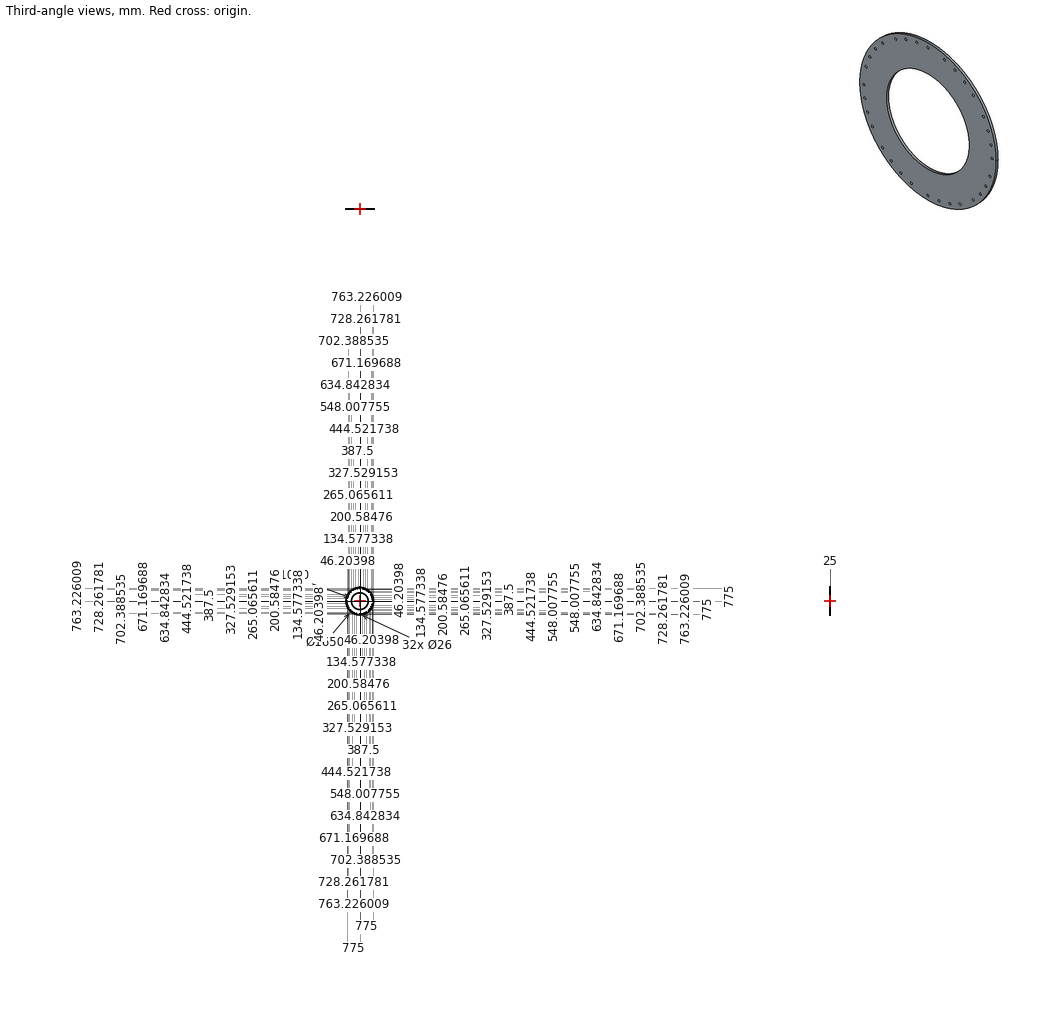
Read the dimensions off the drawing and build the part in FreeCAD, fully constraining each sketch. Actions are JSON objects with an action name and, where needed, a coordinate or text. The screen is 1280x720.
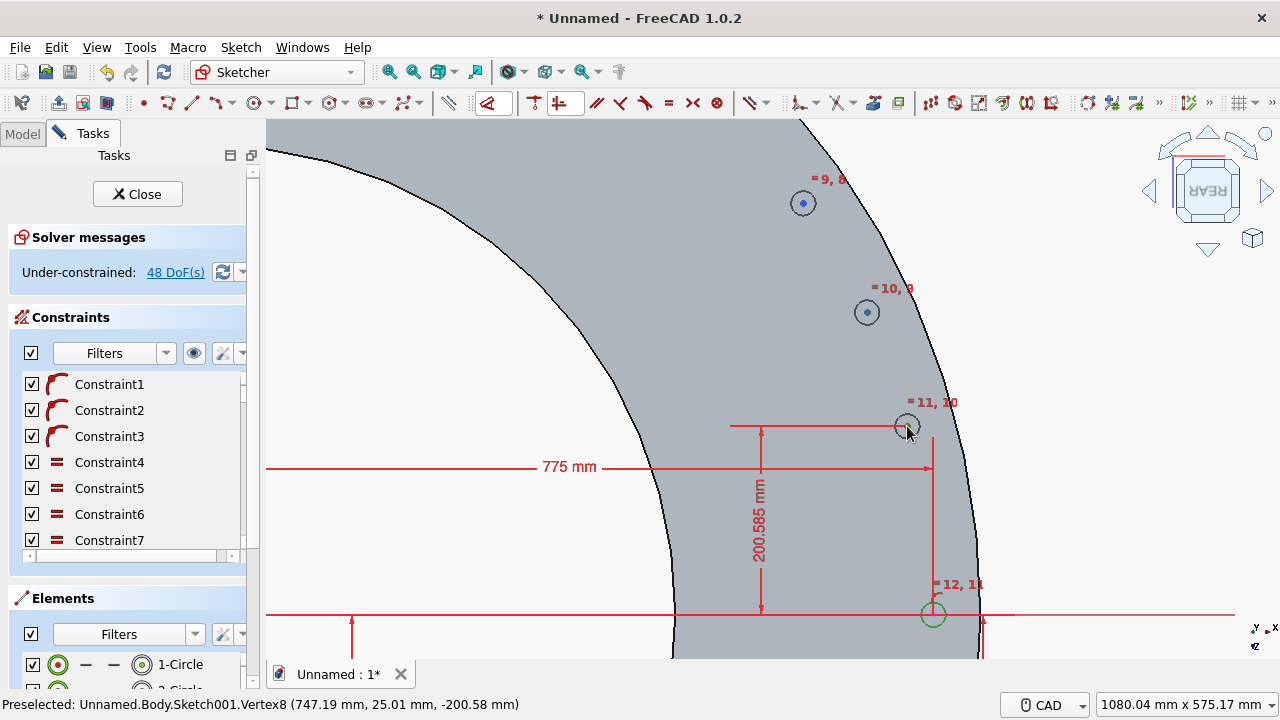
{"action": "key", "text": "l"}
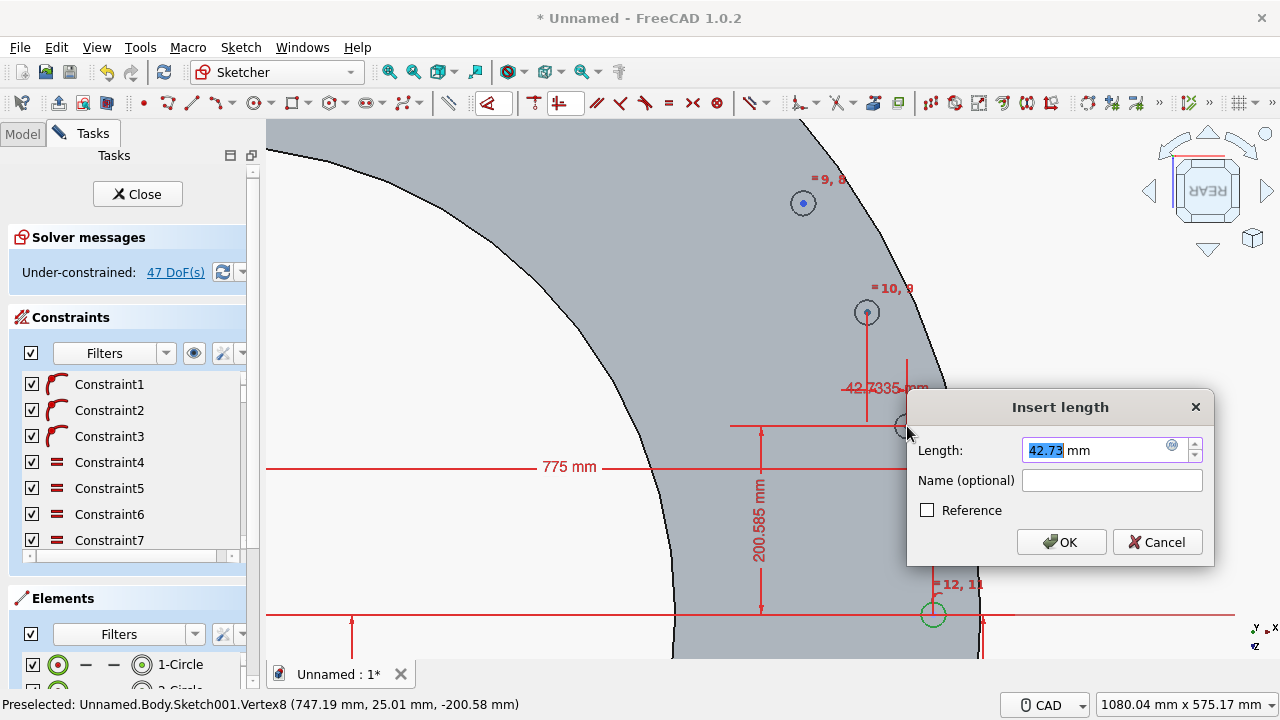
{"action": "type", "text": "46.20398"}
{"action": "key", "text": "Return"}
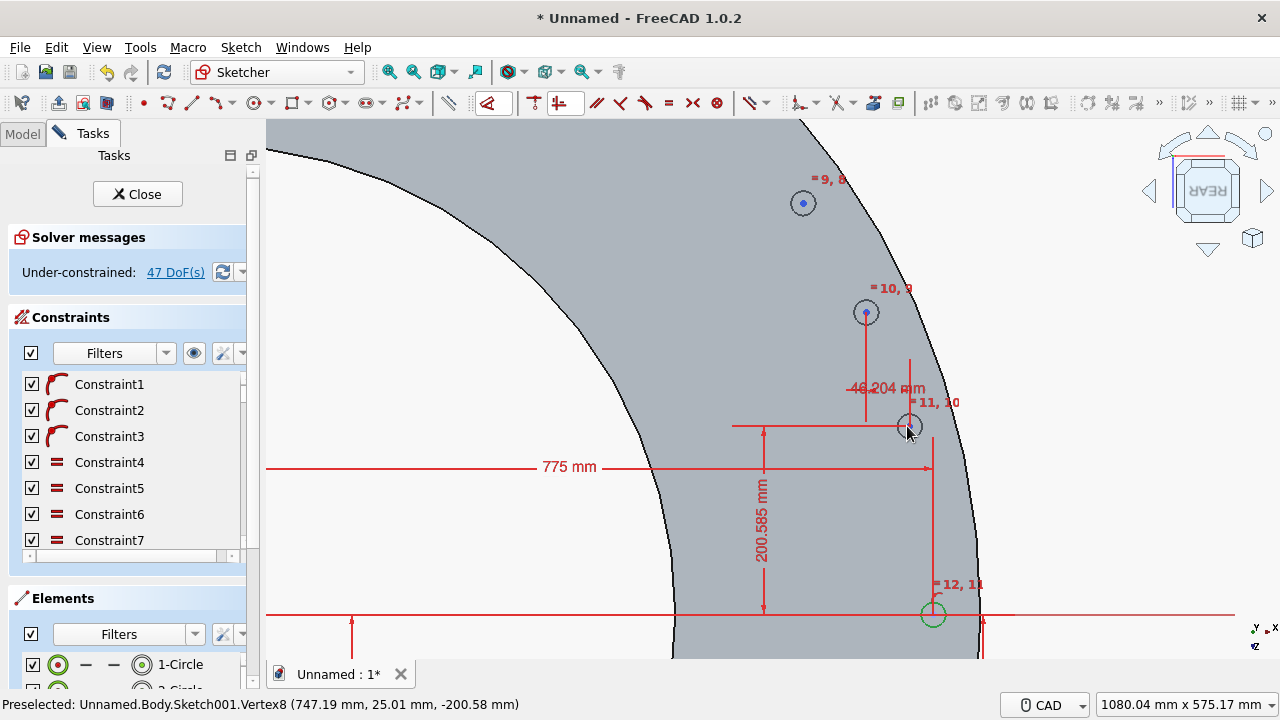
{"action": "scroll", "coordinate": [868, 315], "scroll_direction": "down", "scroll_amount": 7}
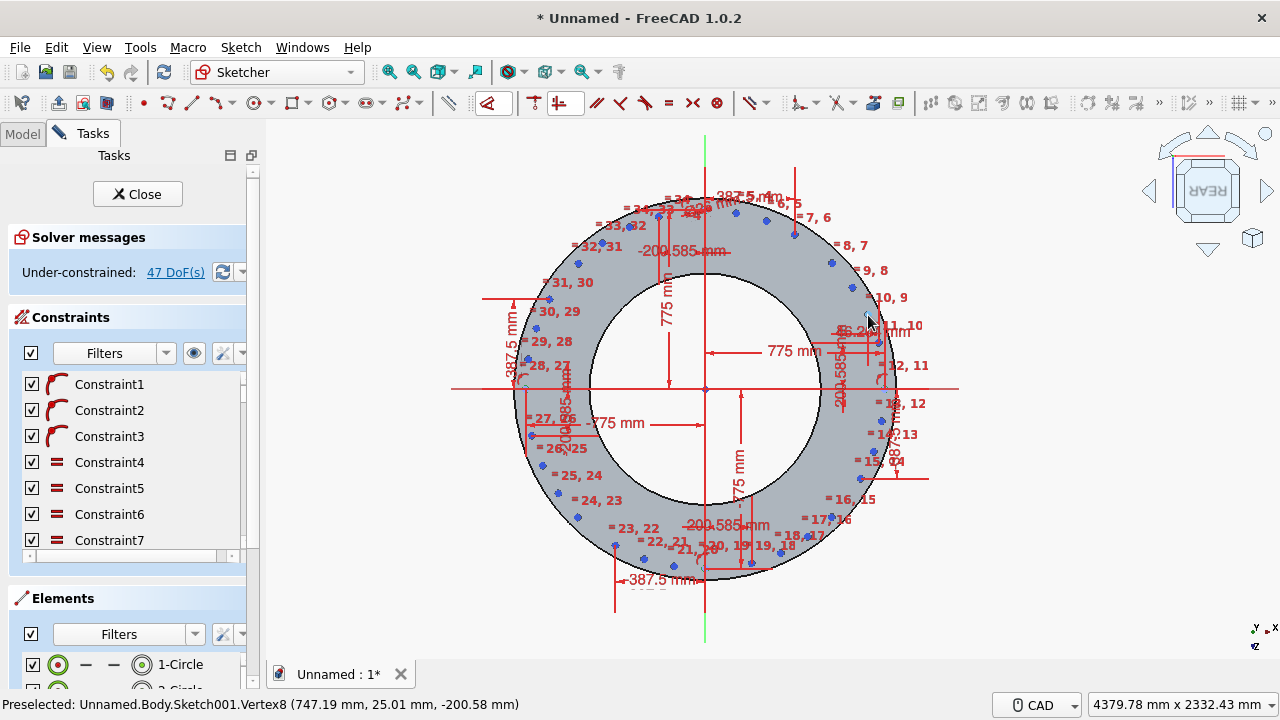
{"action": "scroll", "coordinate": [781, 553], "scroll_direction": "up", "scroll_amount": 7}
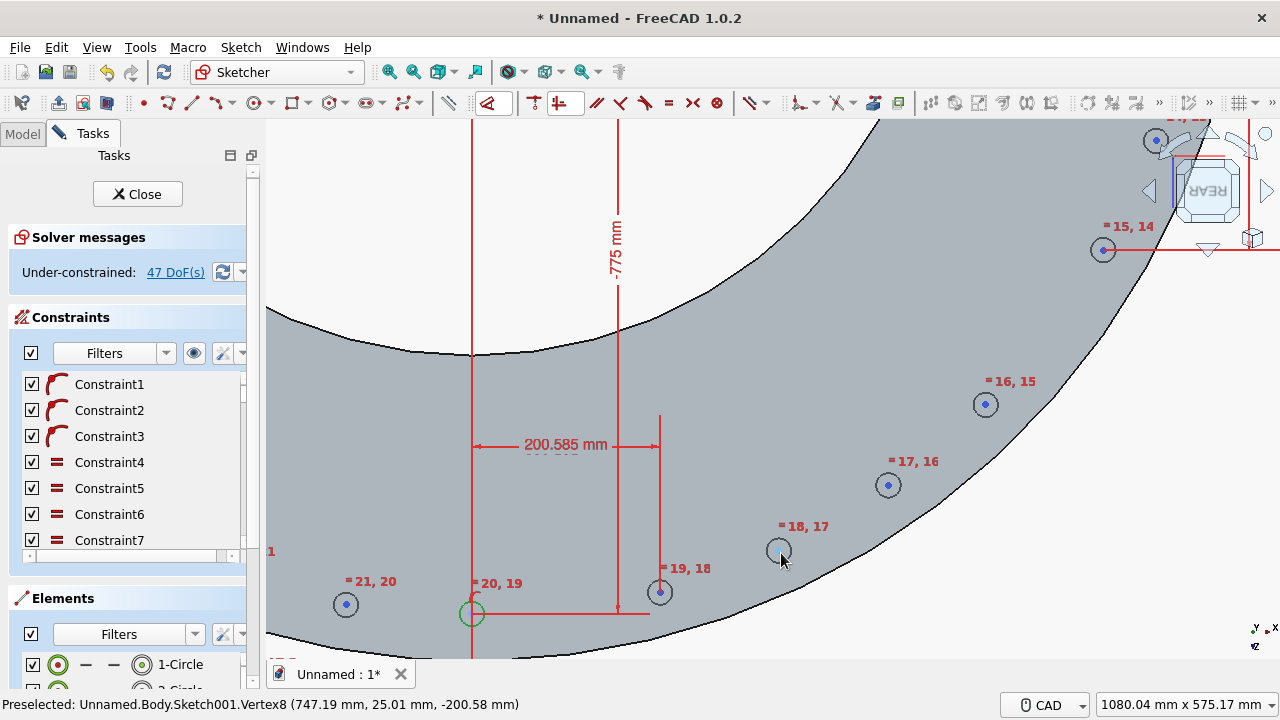
{"action": "left_click", "coordinate": [779, 551]}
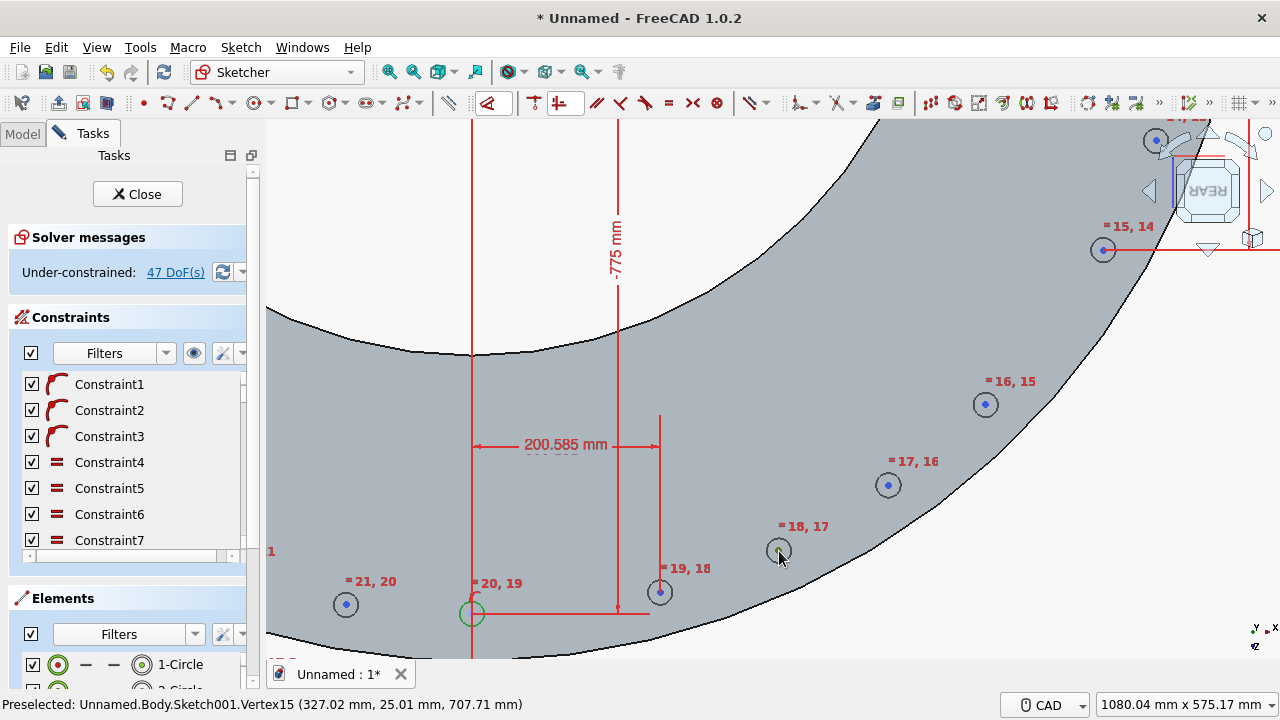
{"action": "left_click", "coordinate": [660, 593]}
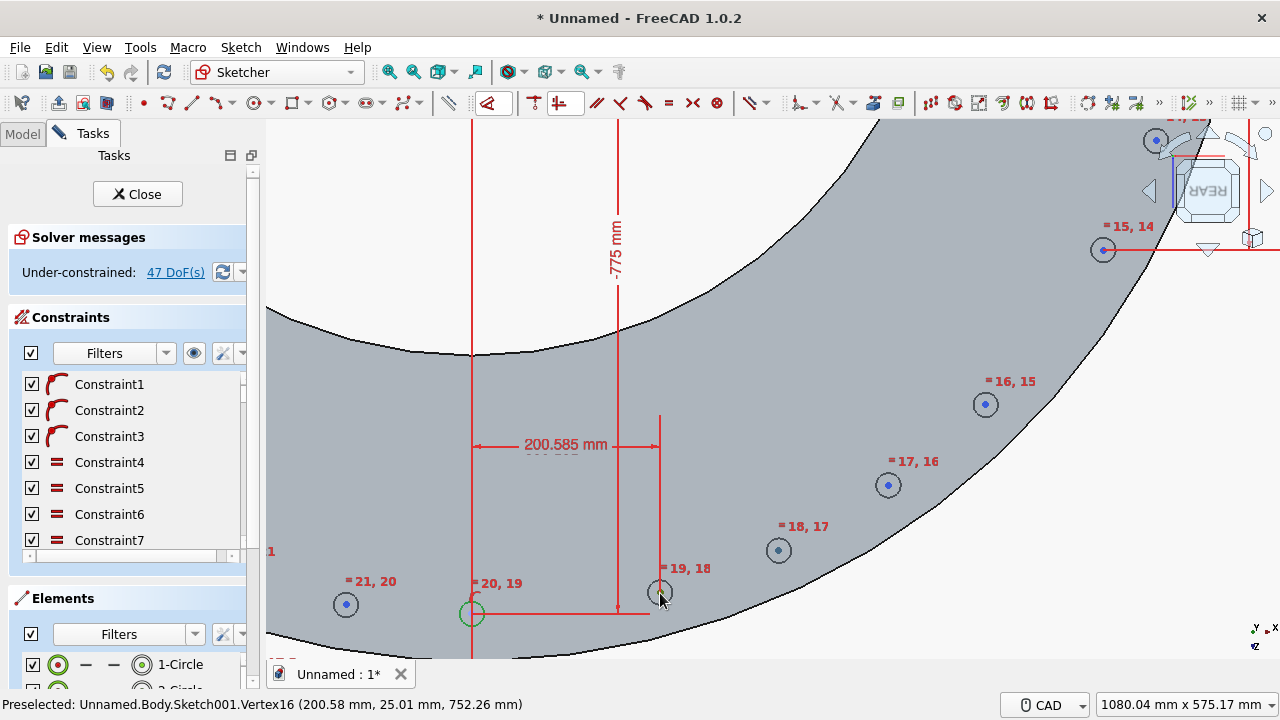
{"action": "key", "text": "i"}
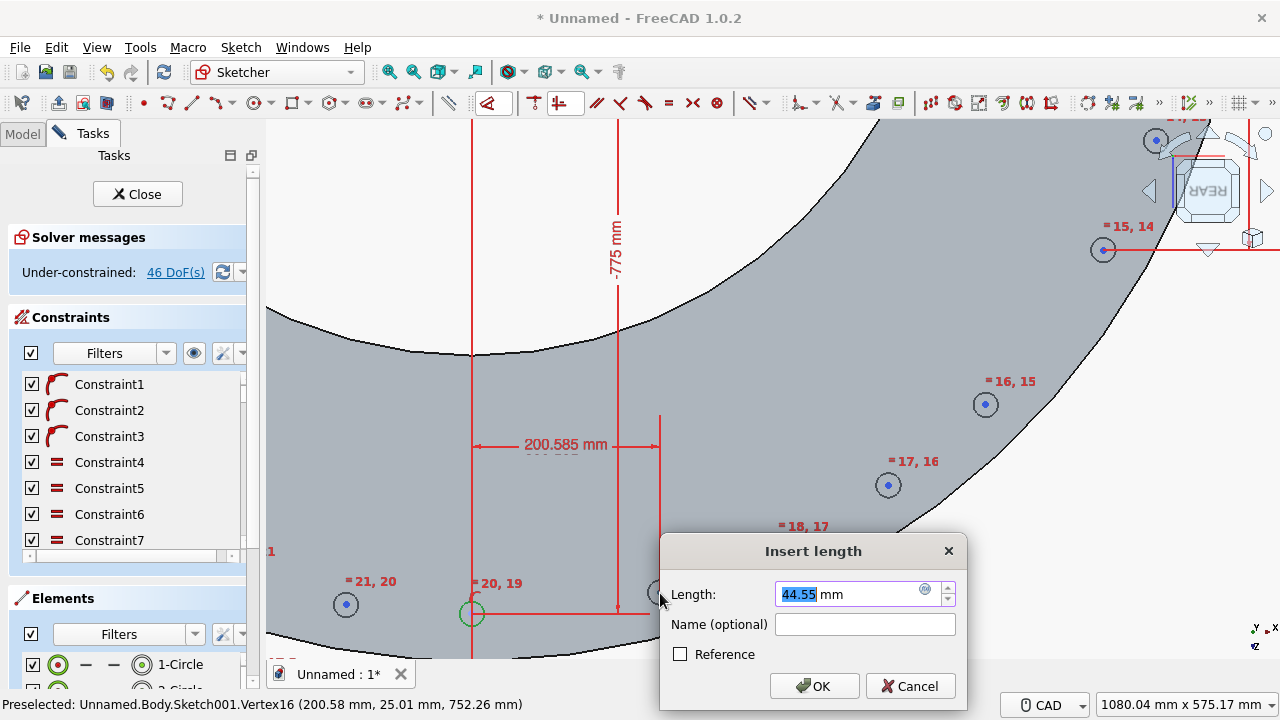
{"action": "type", "text": "46.20398"}
{"action": "key", "text": "Return"}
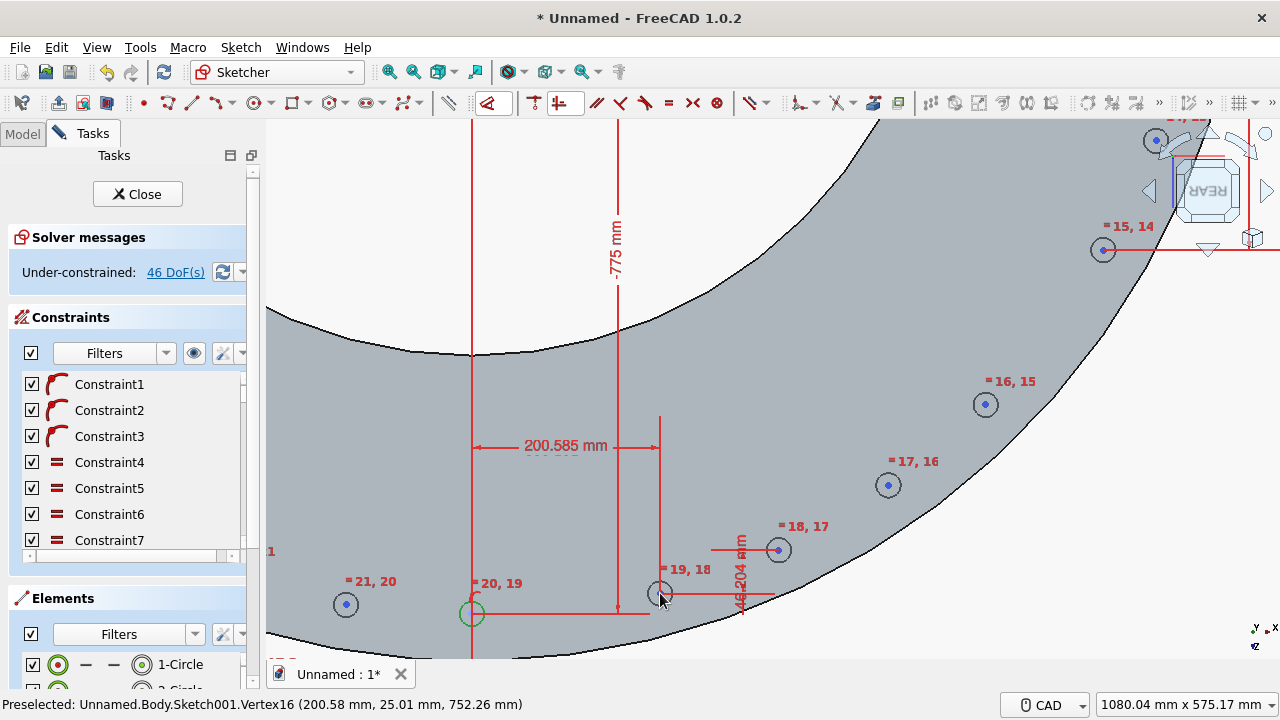
{"action": "scroll", "coordinate": [781, 554], "scroll_direction": "down", "scroll_amount": 7}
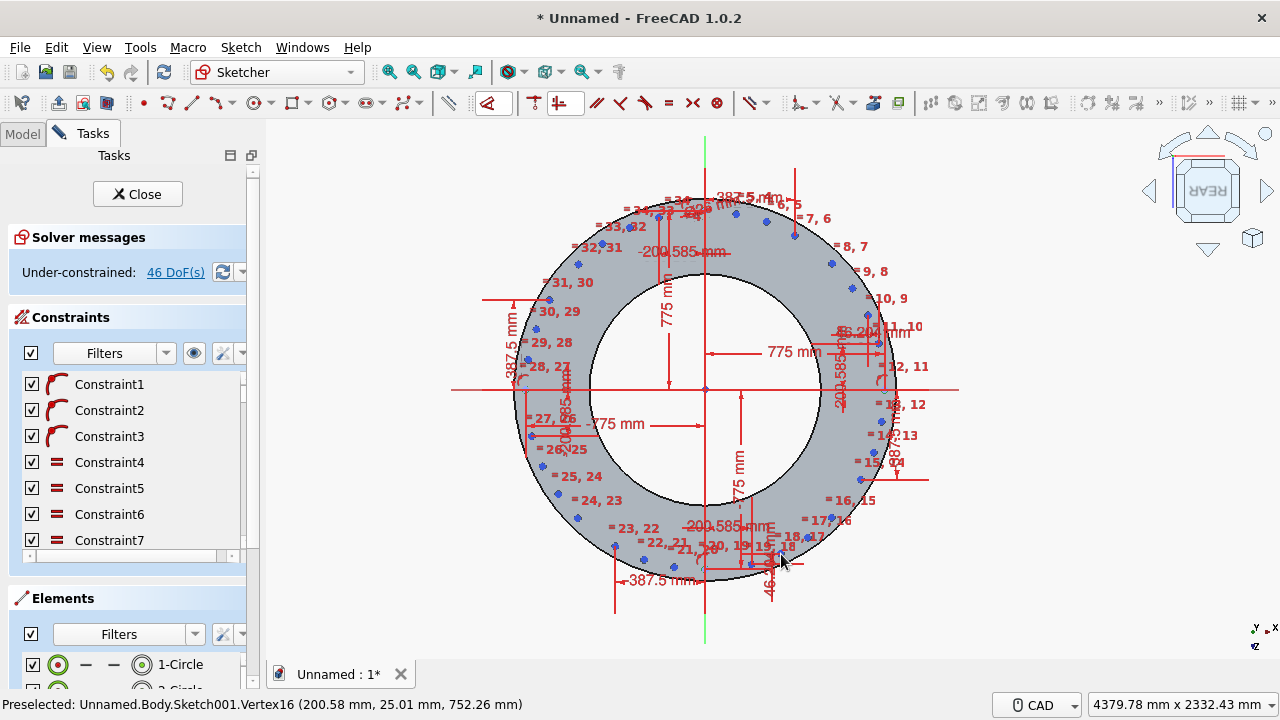
{"action": "scroll", "coordinate": [543, 466], "scroll_direction": "up", "scroll_amount": 7}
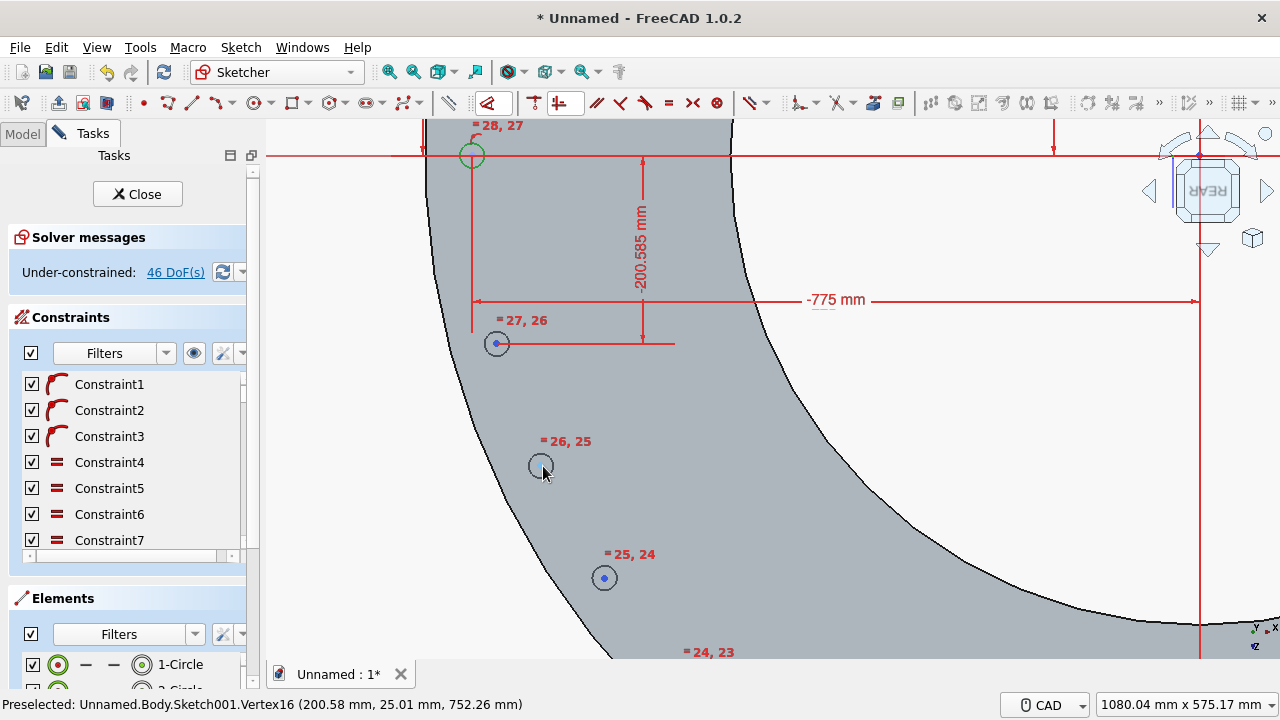
{"action": "left_click", "coordinate": [541, 466]}